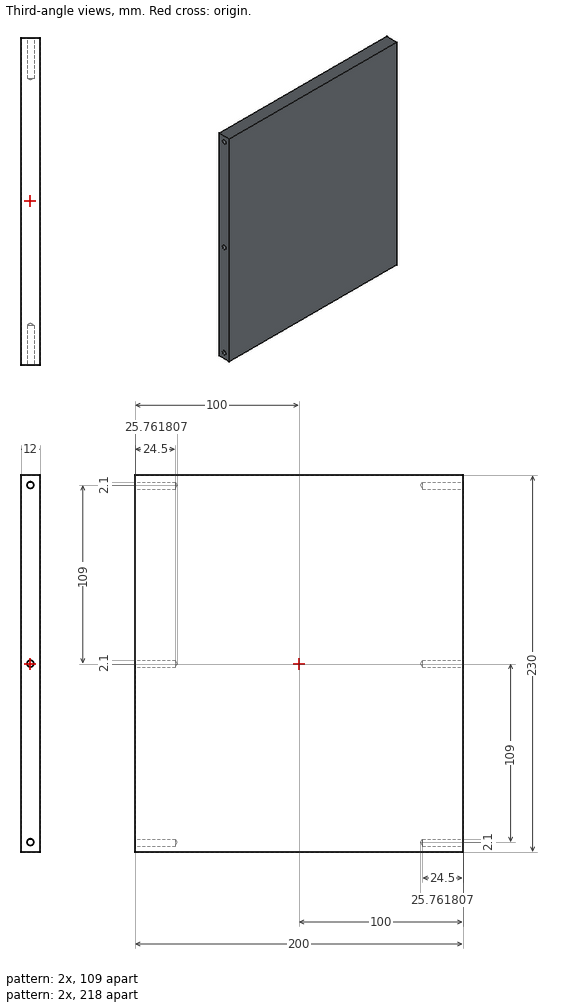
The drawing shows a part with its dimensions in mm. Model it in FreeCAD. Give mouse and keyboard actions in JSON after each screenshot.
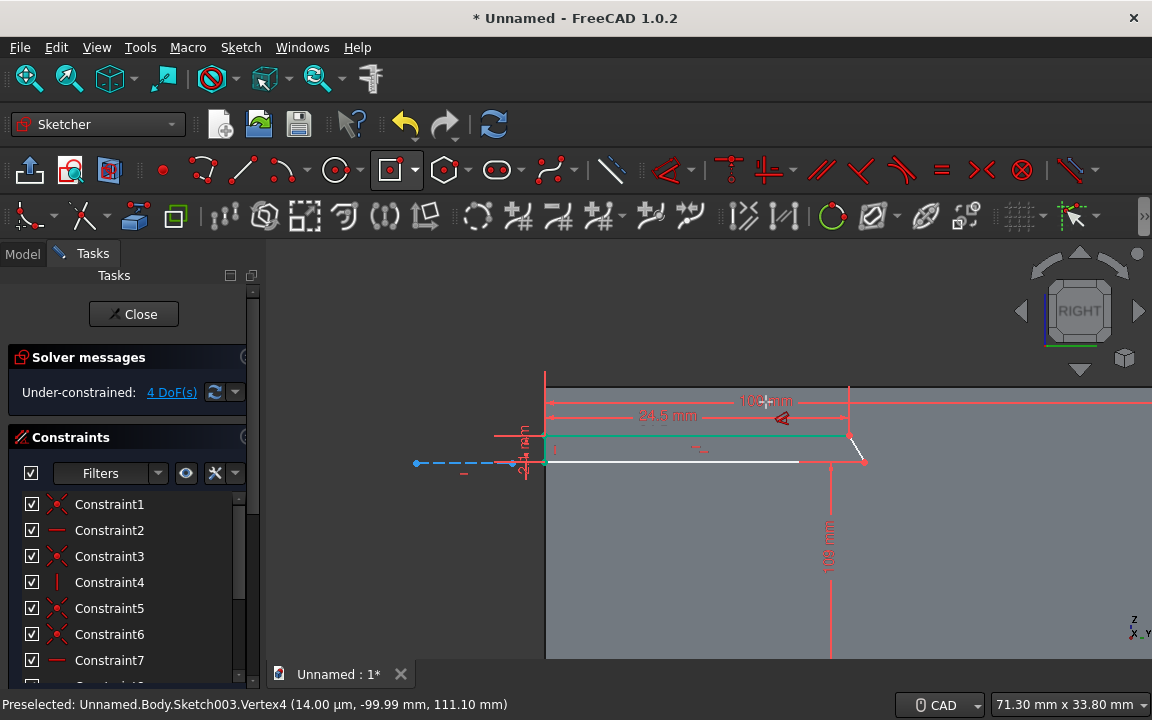
{"action": "left_click", "coordinate": [513, 463]}
{"action": "left_click", "coordinate": [479, 547]}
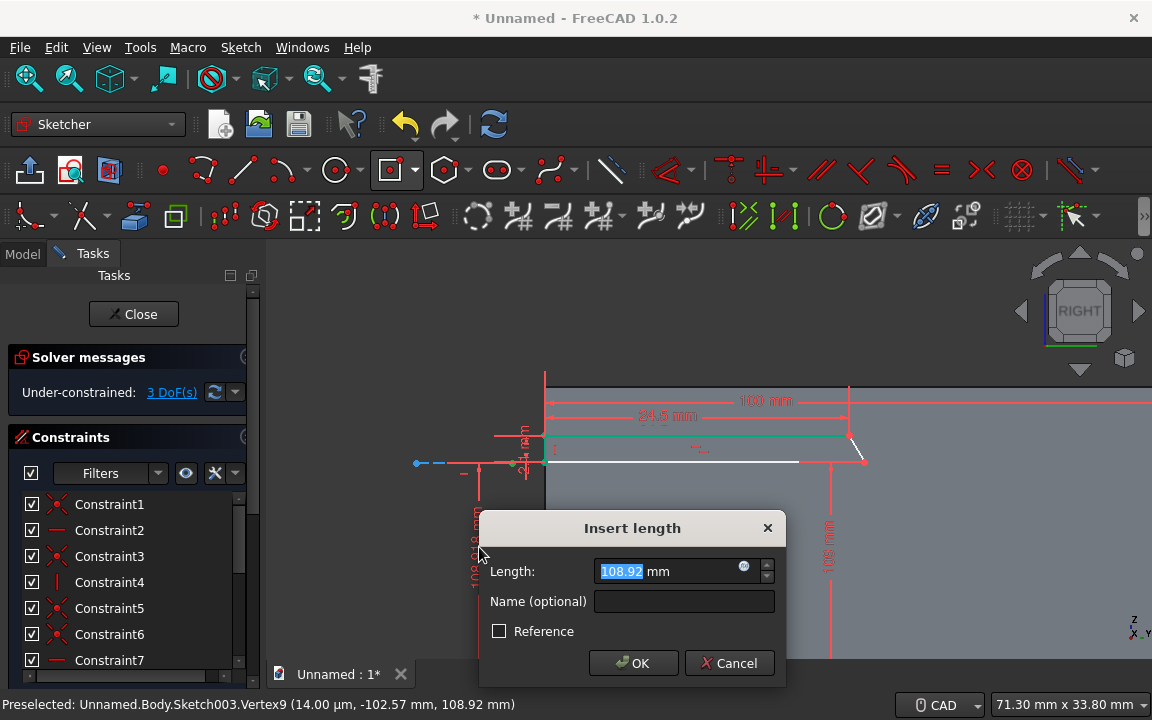
{"action": "type", "text": "109"}
{"action": "key", "text": "Return"}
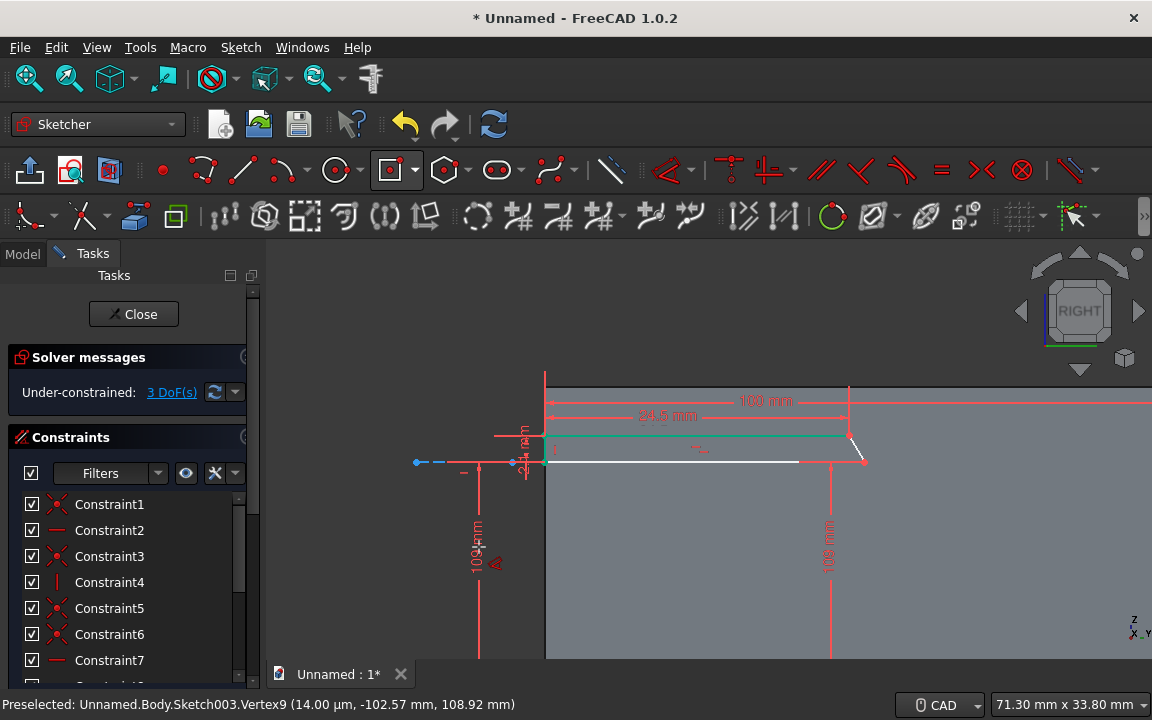
{"action": "left_click", "coordinate": [641, 462]}
{"action": "left_click", "coordinate": [705, 496]}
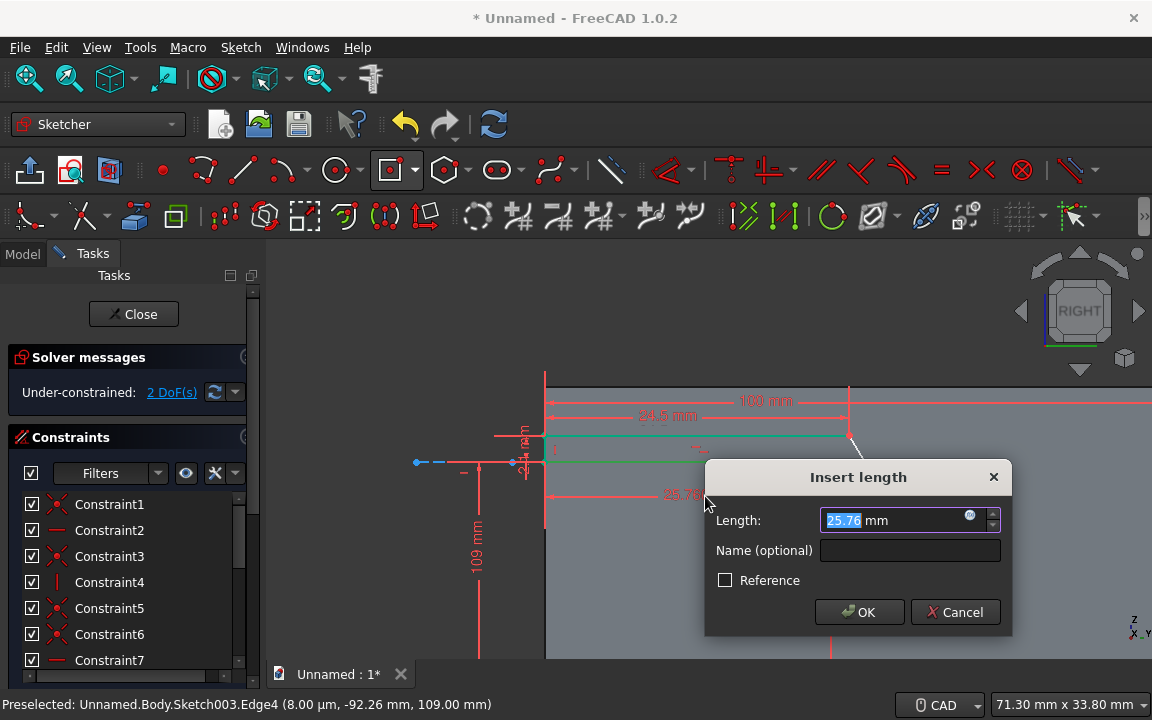
{"action": "type", "text": "25.761807"}
{"action": "key", "text": "Return"}
{"action": "key", "text": "Escape"}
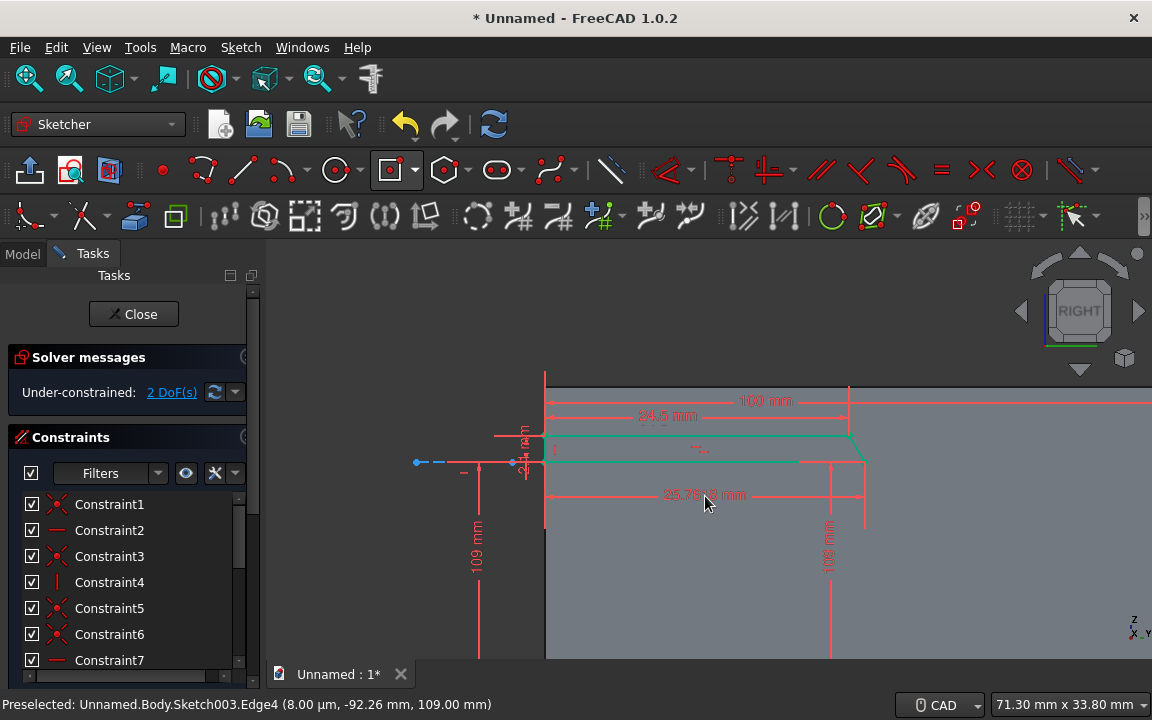
{"action": "left_click", "coordinate": [134, 314]}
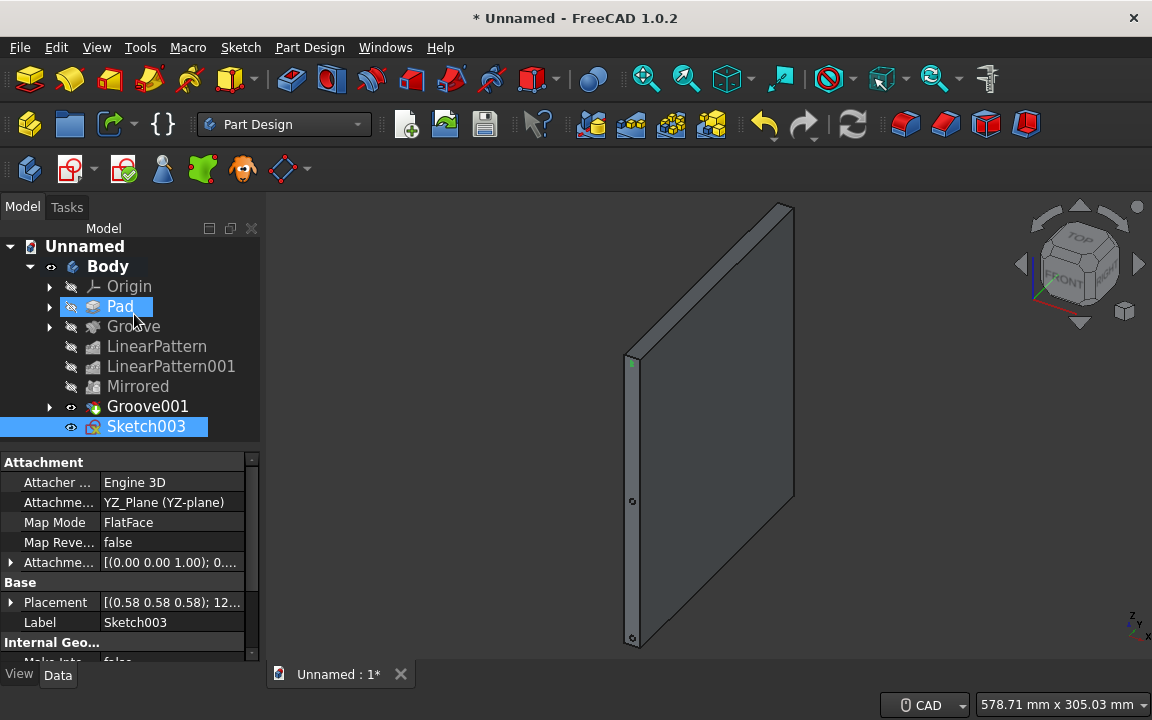
{"action": "left_click", "coordinate": [372, 80]}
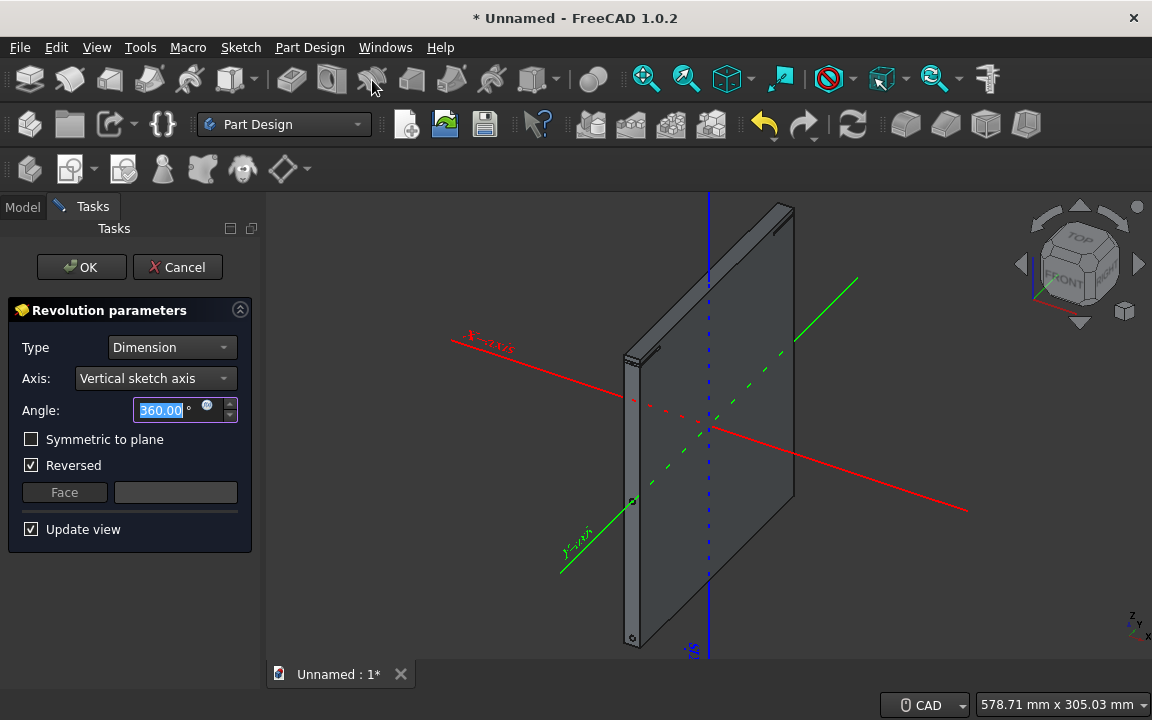
{"action": "left_click", "coordinate": [156, 378]}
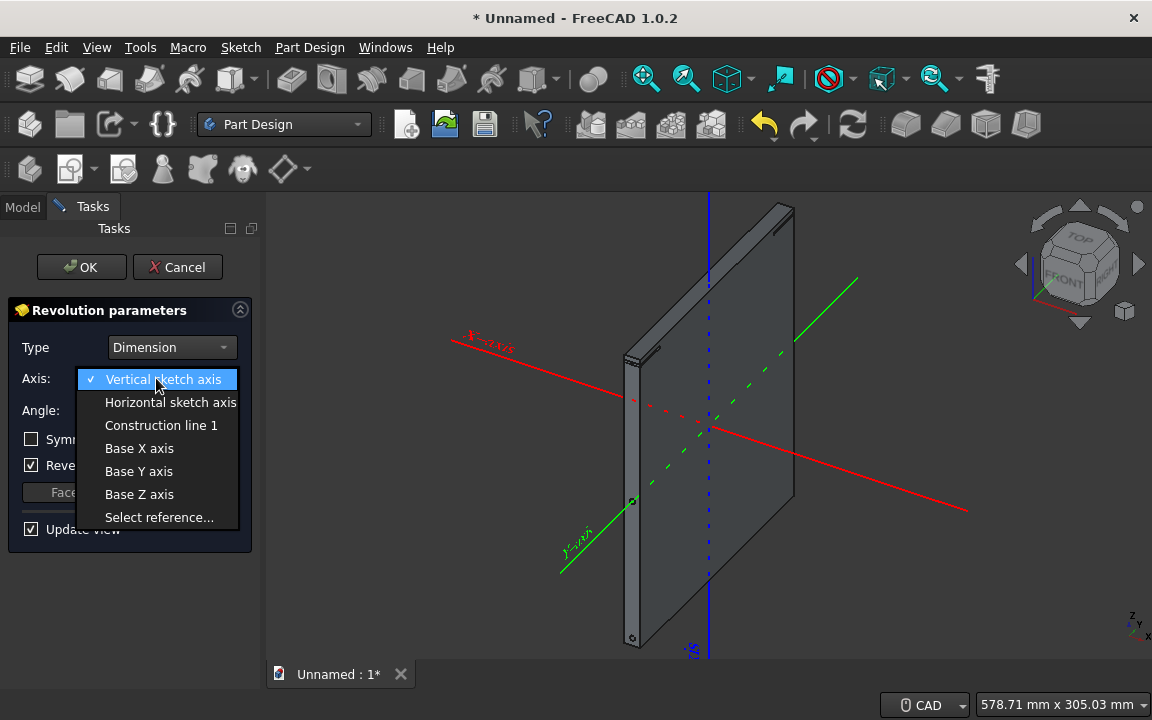
{"action": "left_click", "coordinate": [156, 426]}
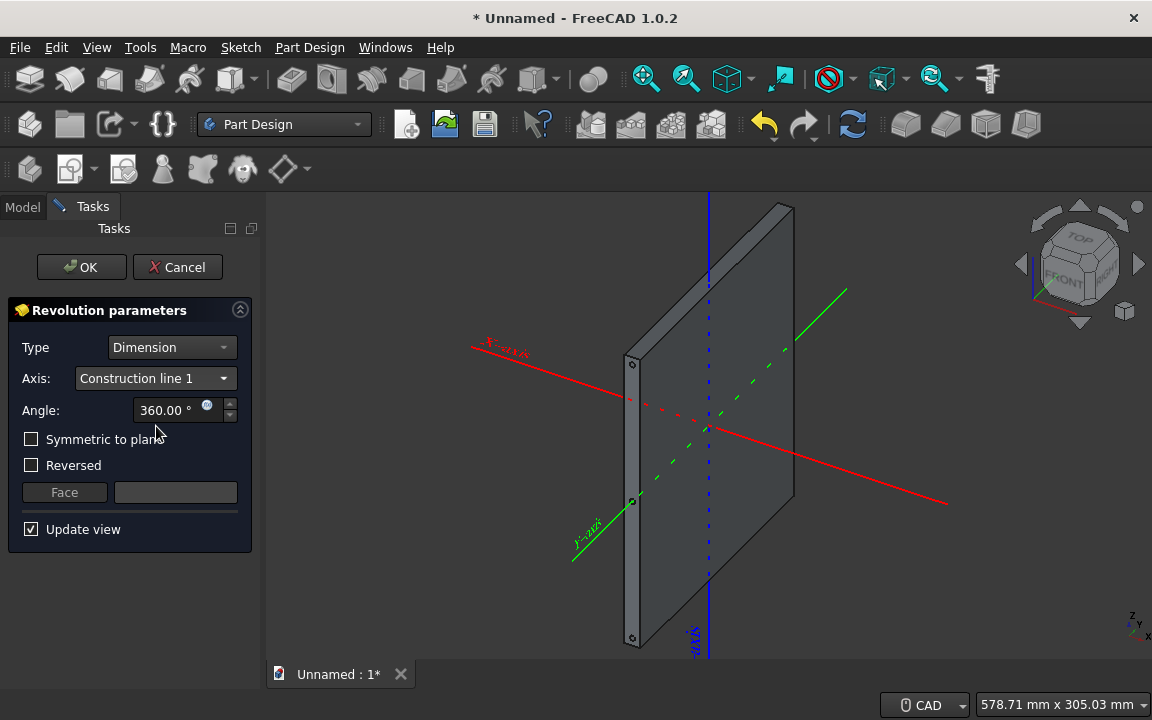
{"action": "left_click", "coordinate": [82, 267]}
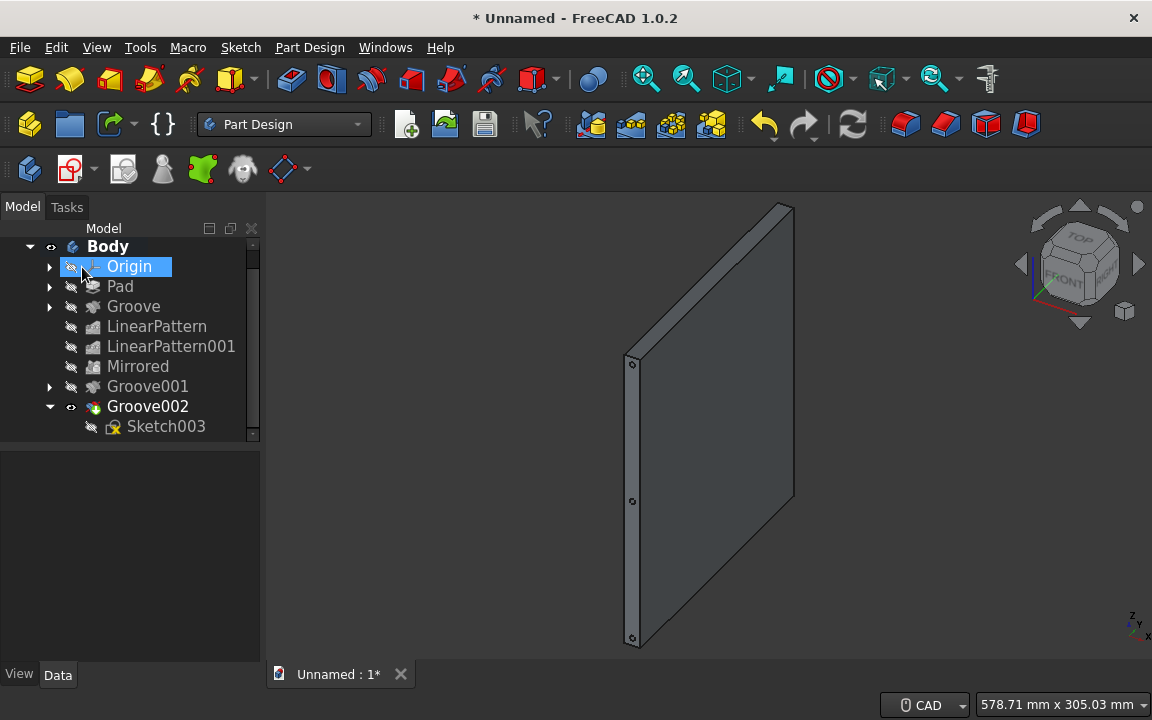
{"action": "key", "text": "0"}